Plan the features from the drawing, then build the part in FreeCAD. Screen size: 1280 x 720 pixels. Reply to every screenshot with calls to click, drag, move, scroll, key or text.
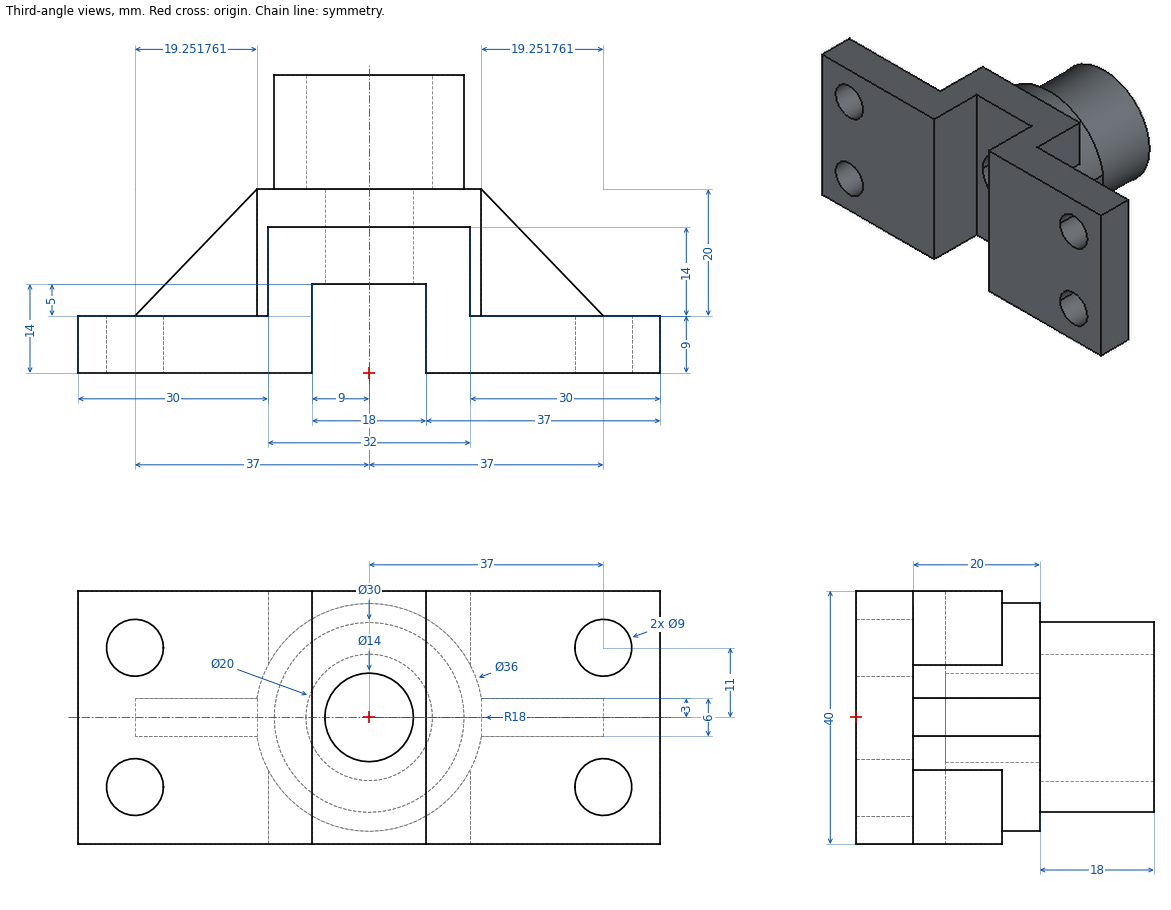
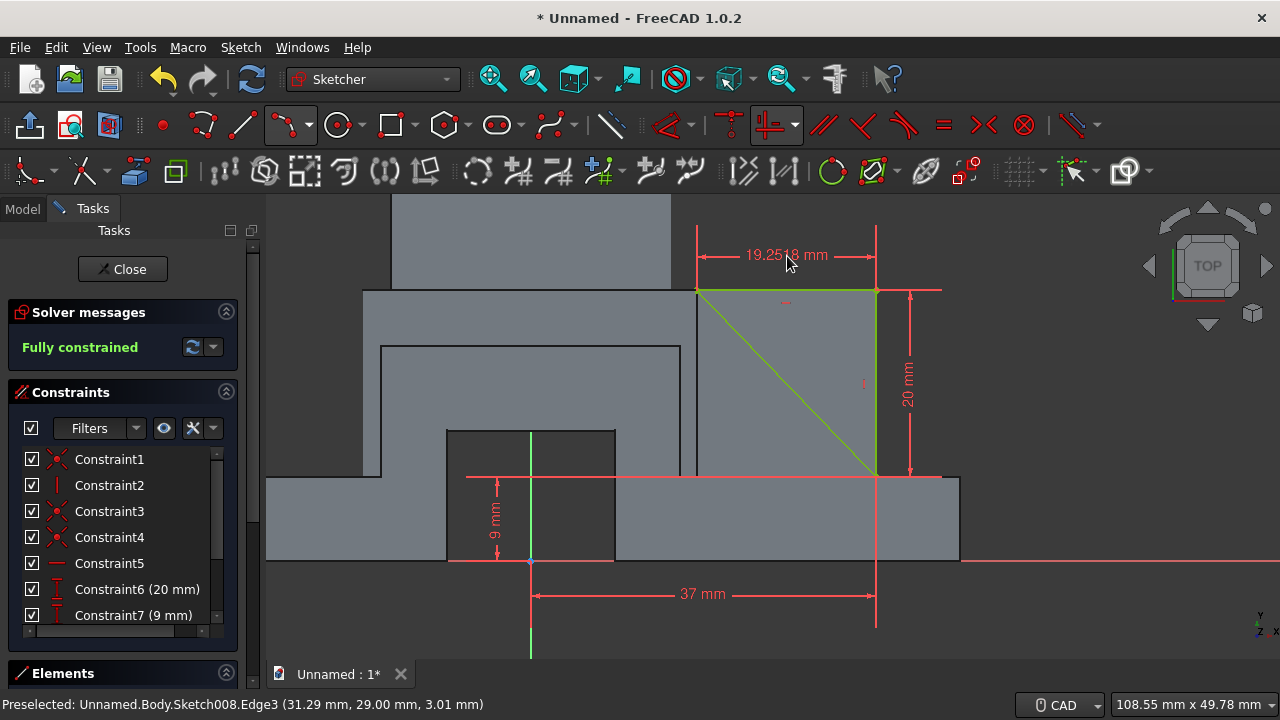
click(123, 269)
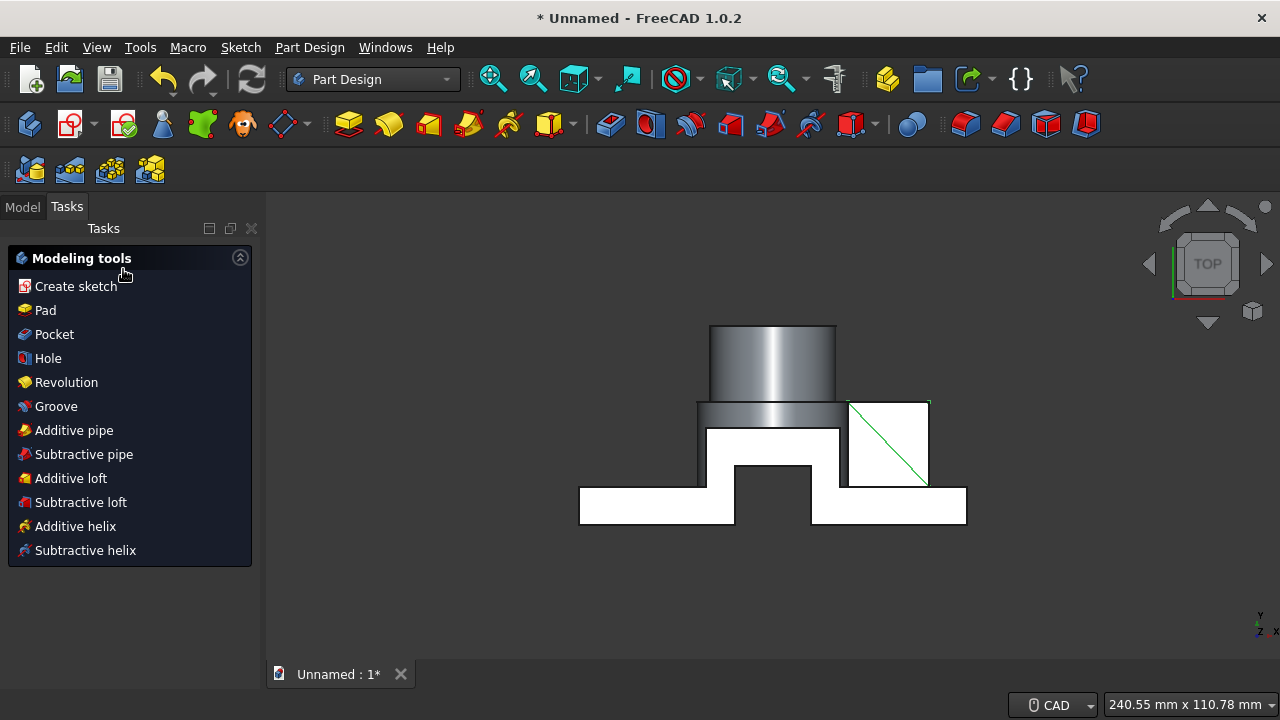
click(612, 124)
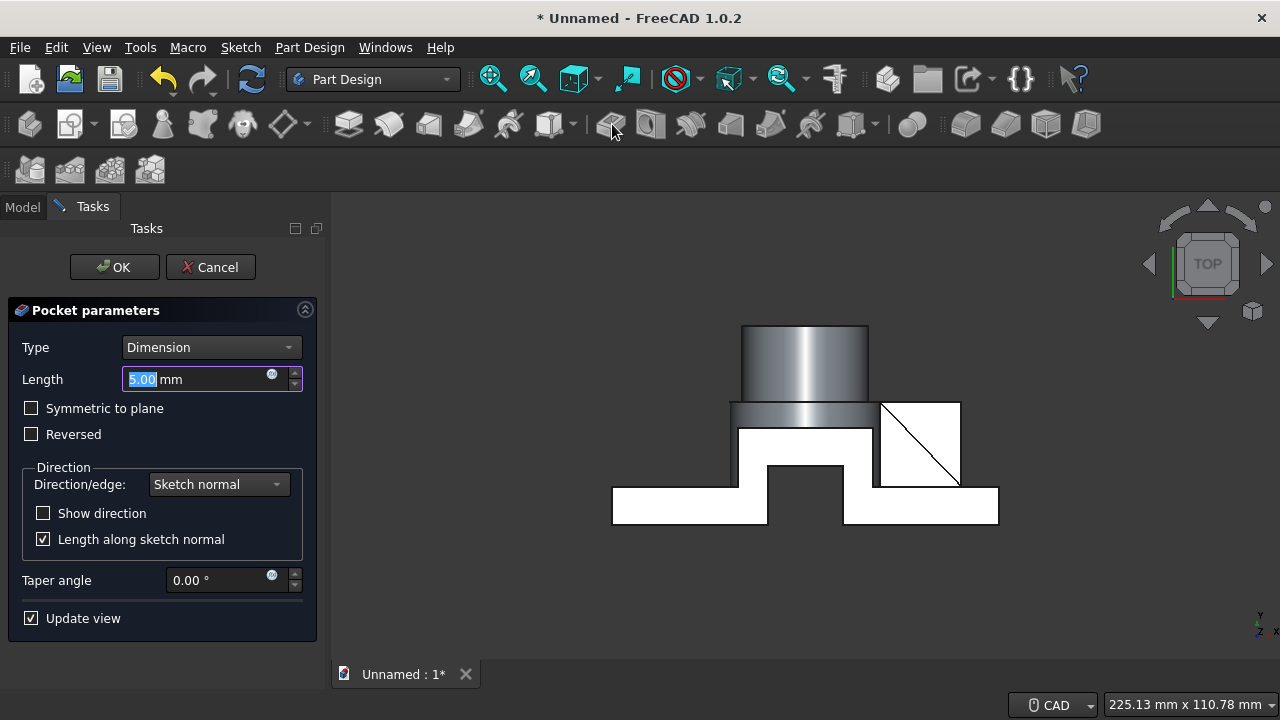
click(212, 348)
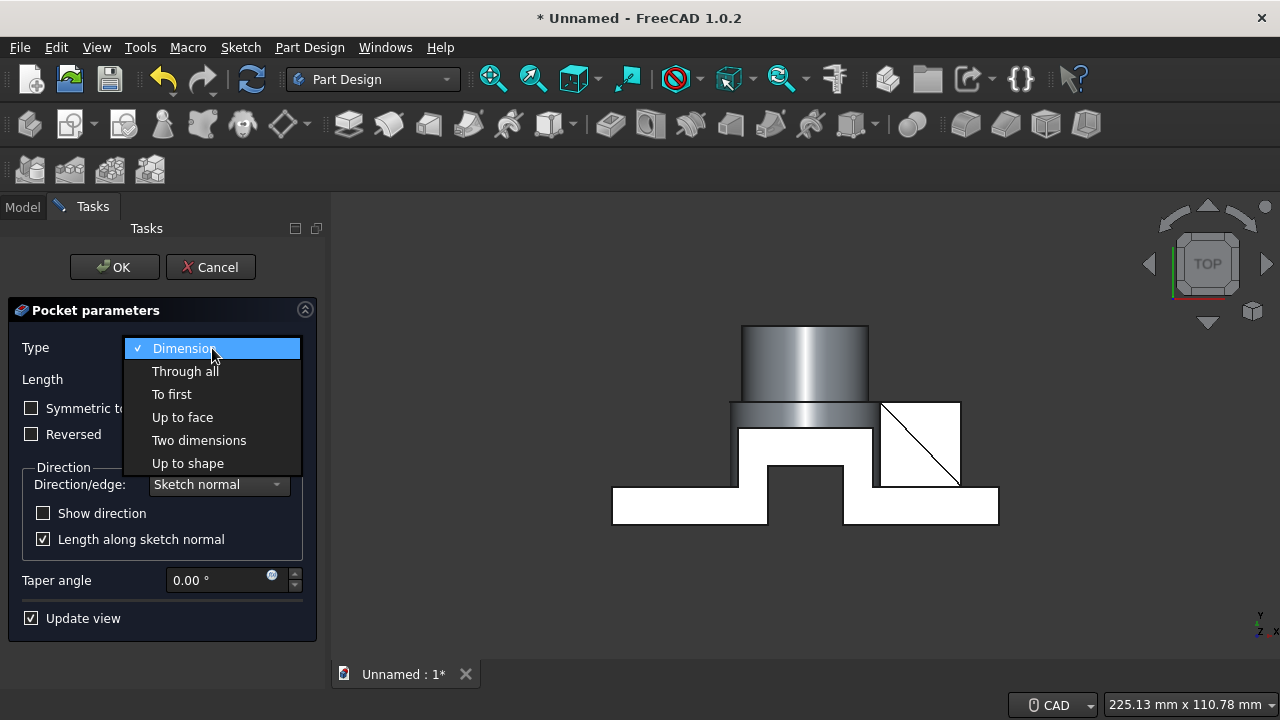
click(212, 372)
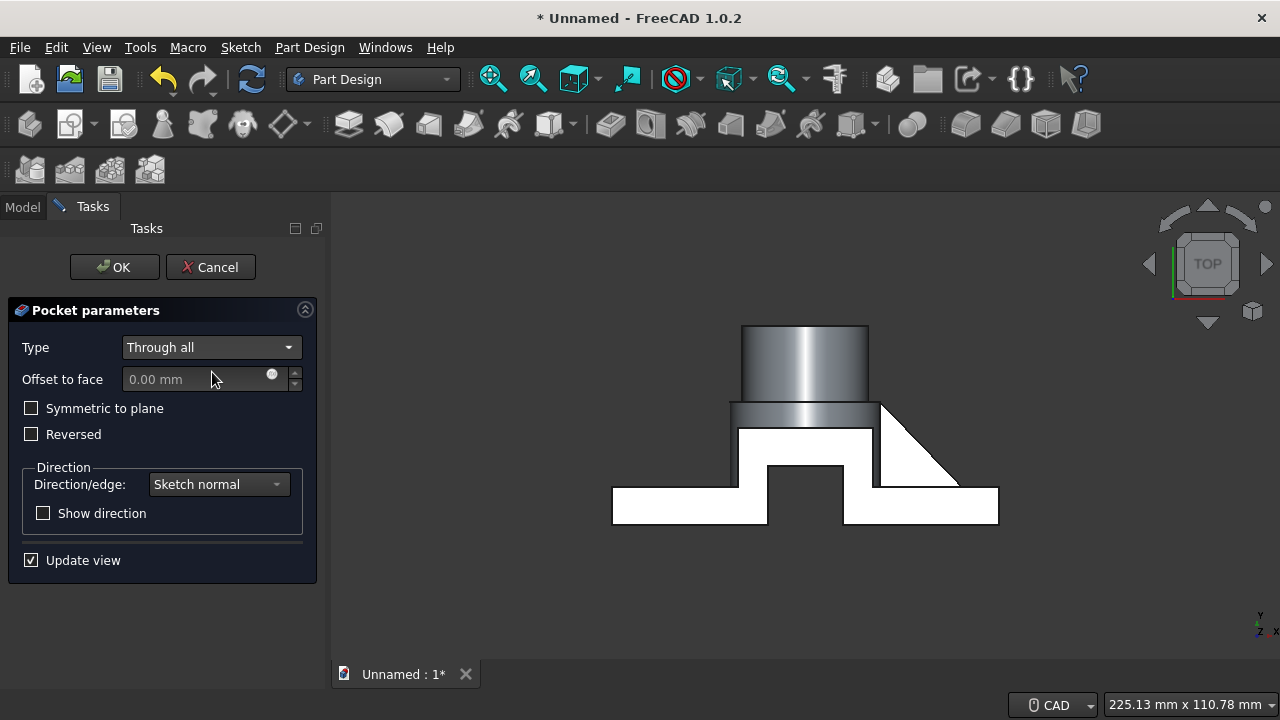
click(115, 267)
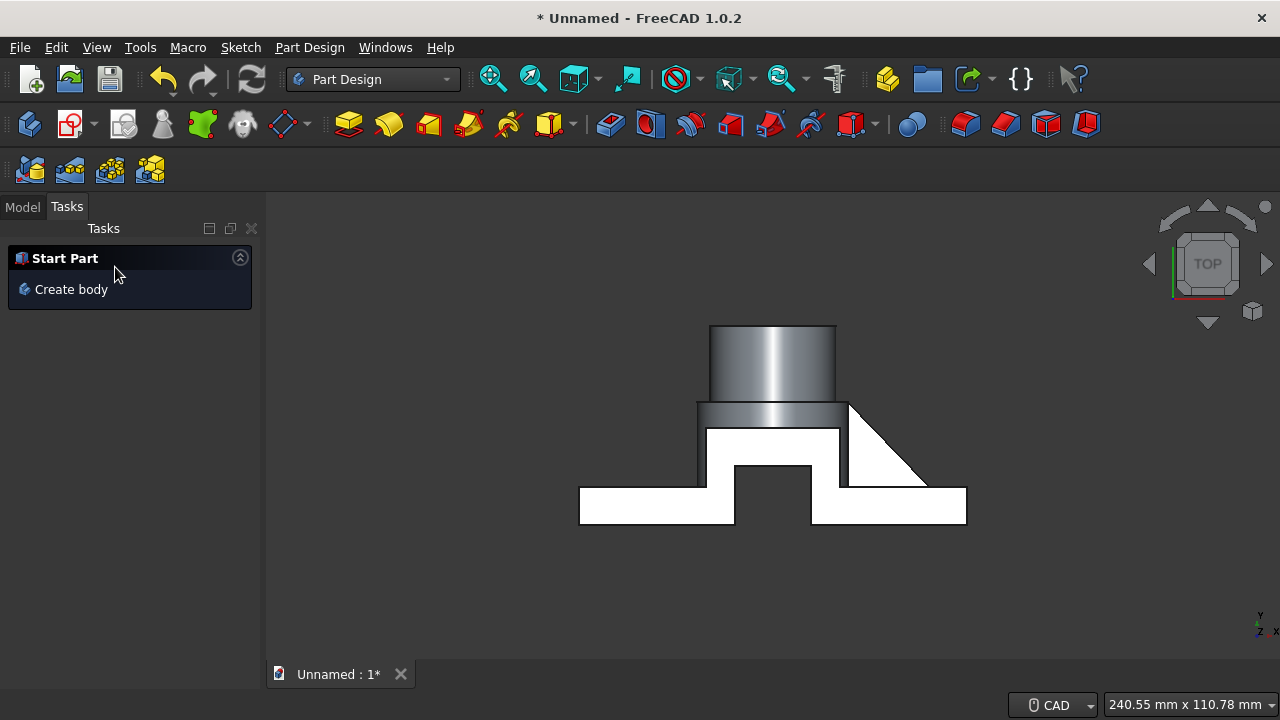
key(v)
key(f)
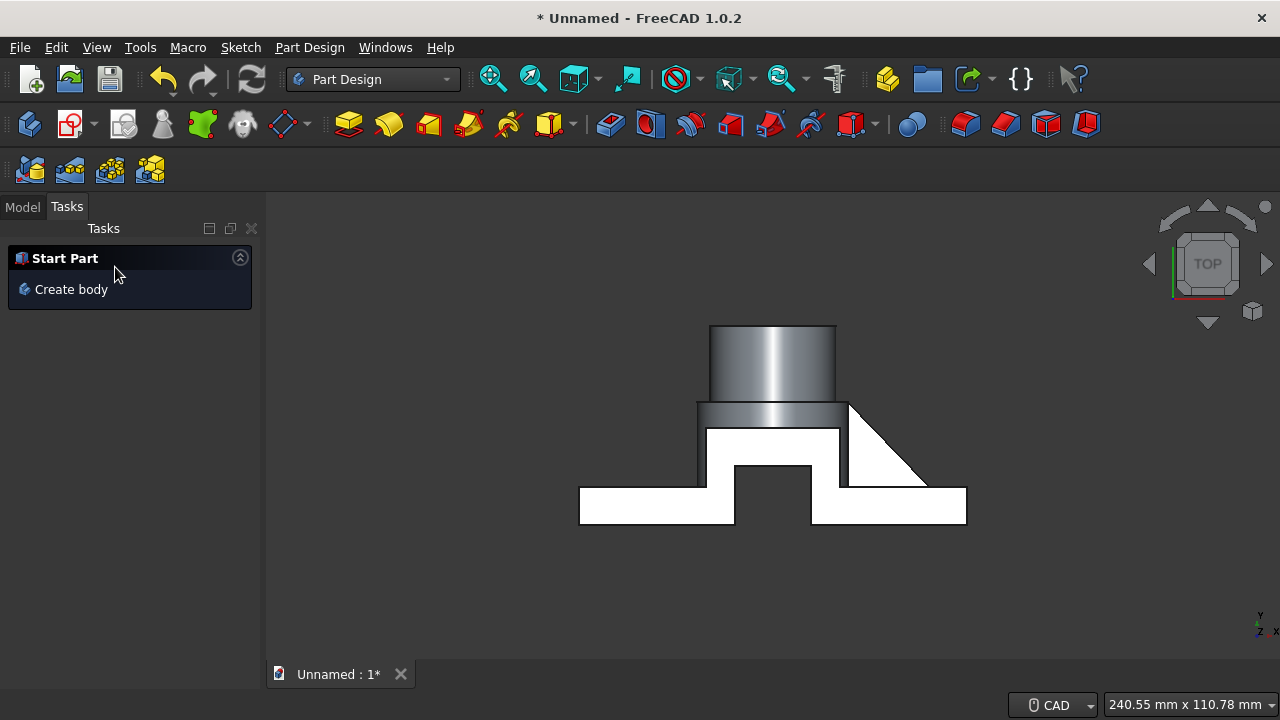
click(23, 206)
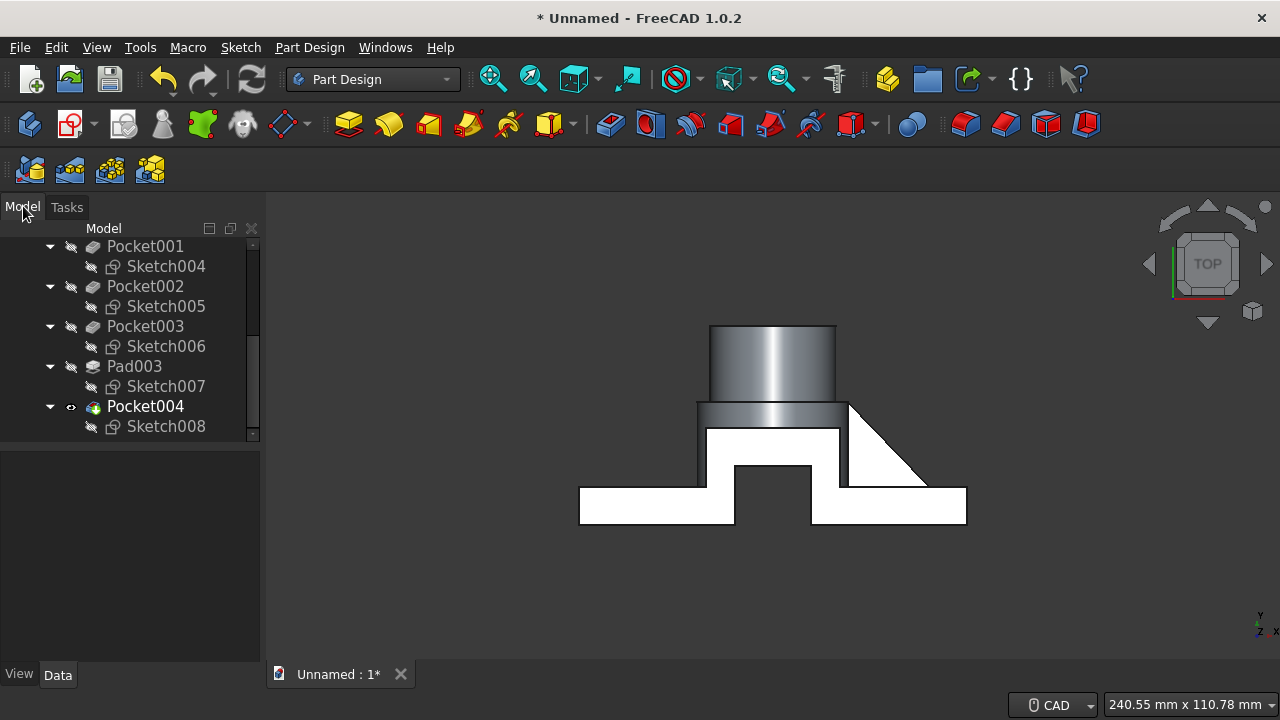
click(116, 327)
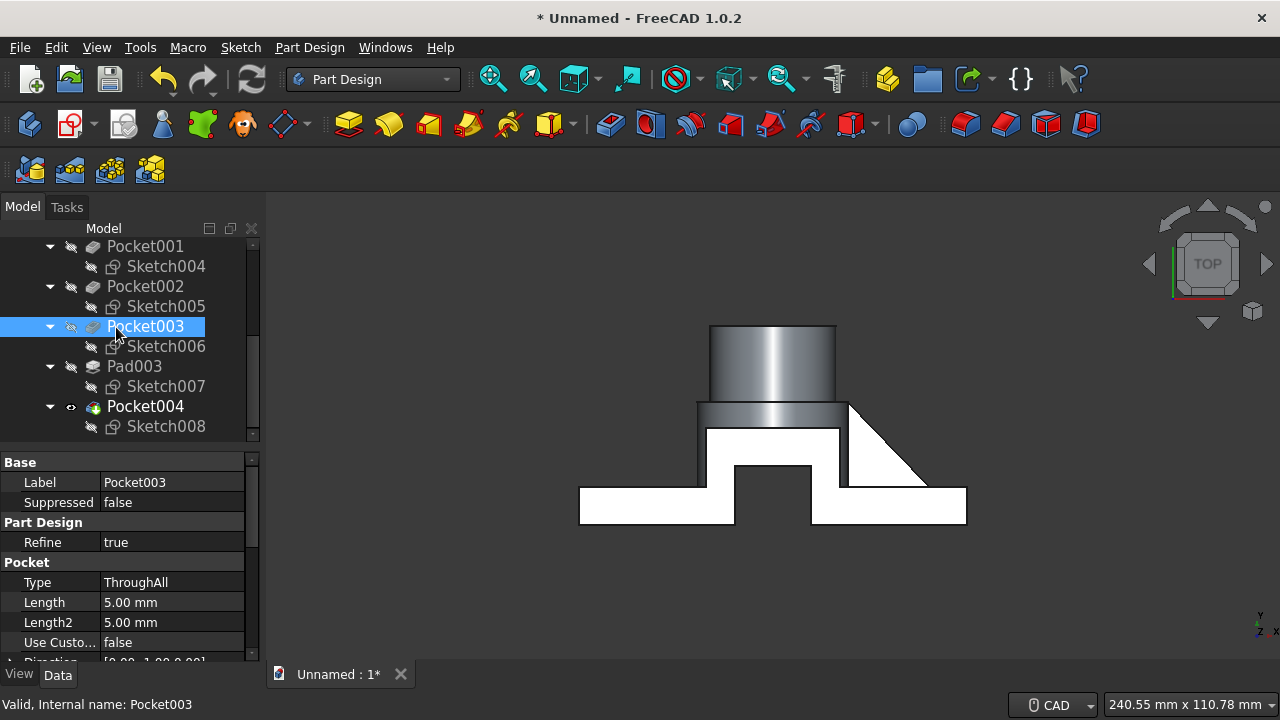
click(116, 367, ctrl)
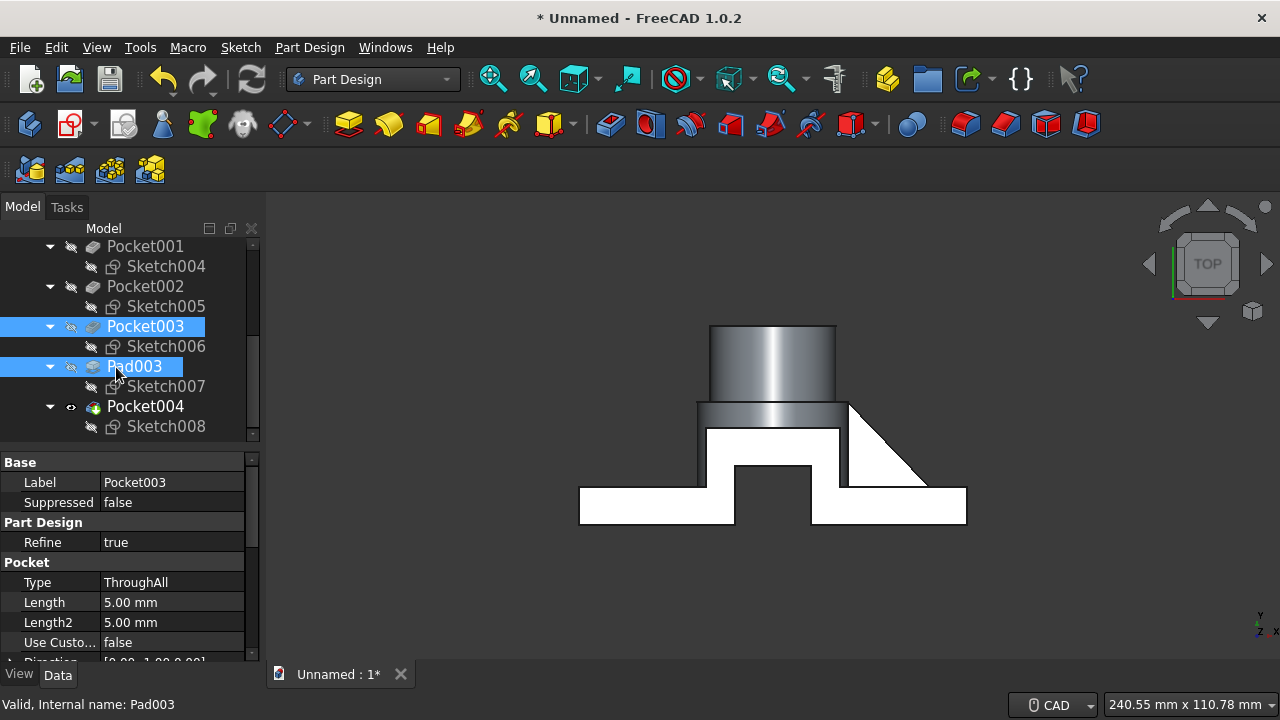
click(30, 170)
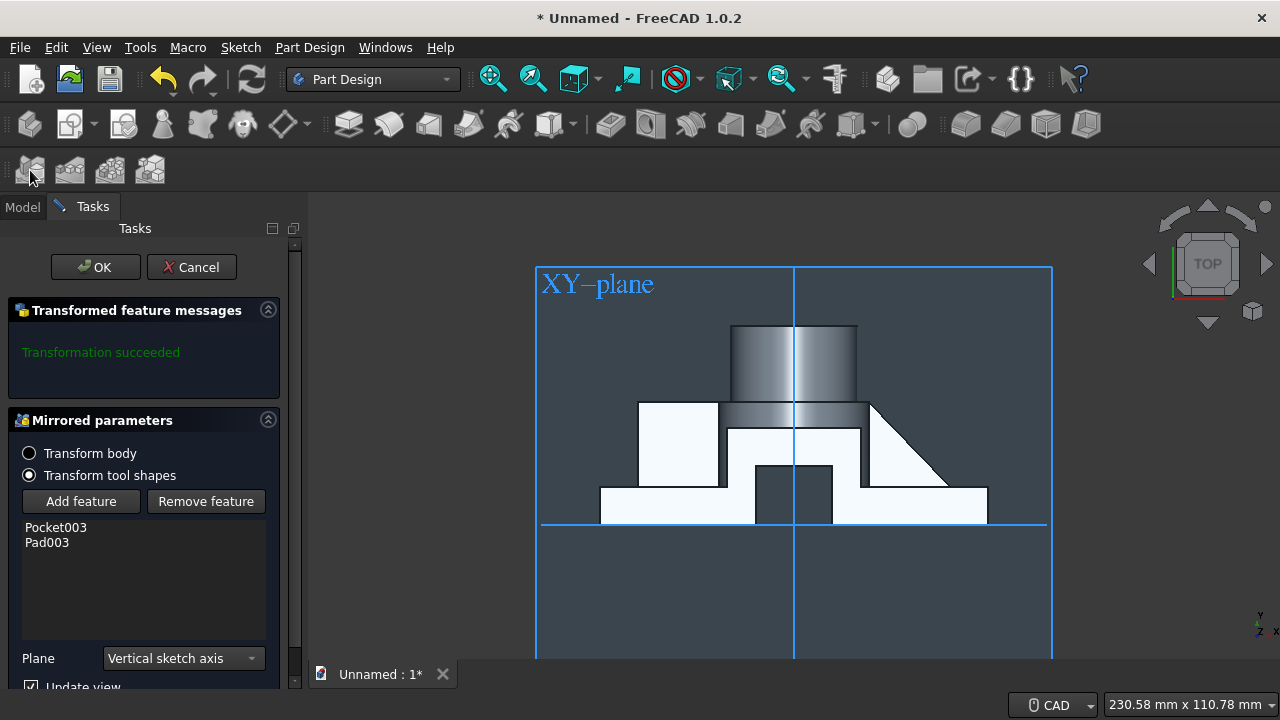
click(184, 658)